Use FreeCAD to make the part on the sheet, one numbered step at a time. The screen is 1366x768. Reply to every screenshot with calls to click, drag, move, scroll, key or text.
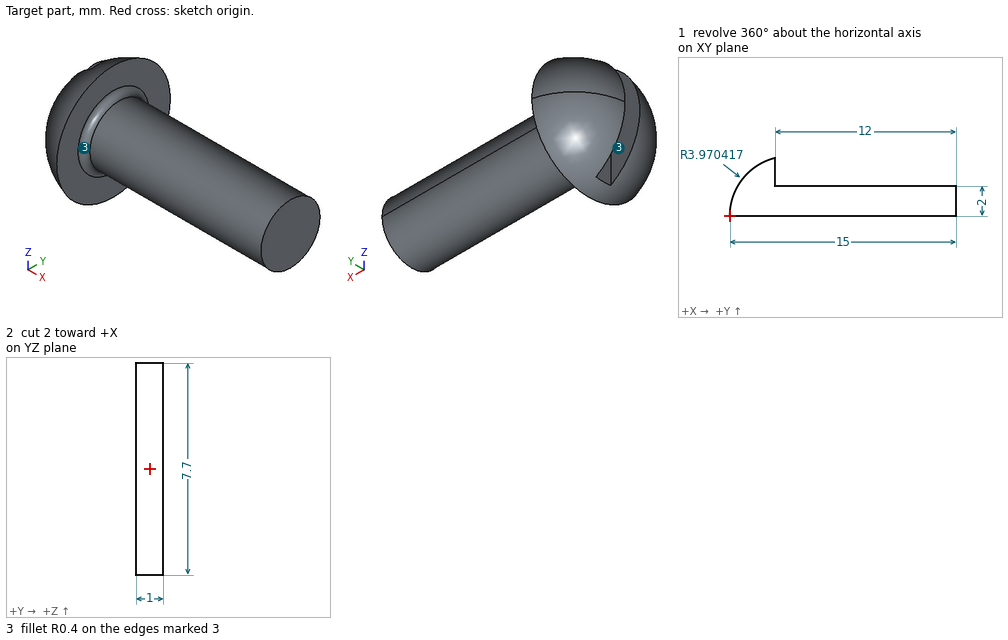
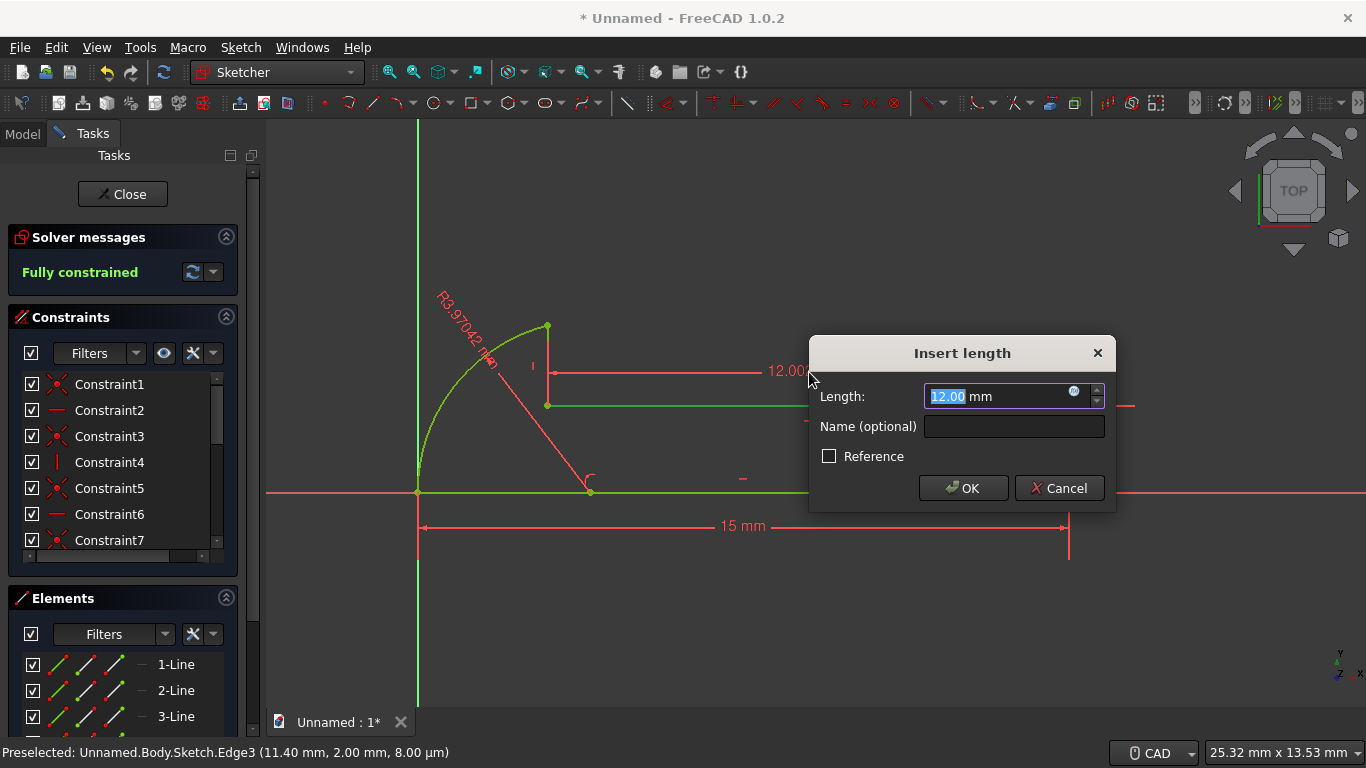
text(12)
key(Return)
key(Escape)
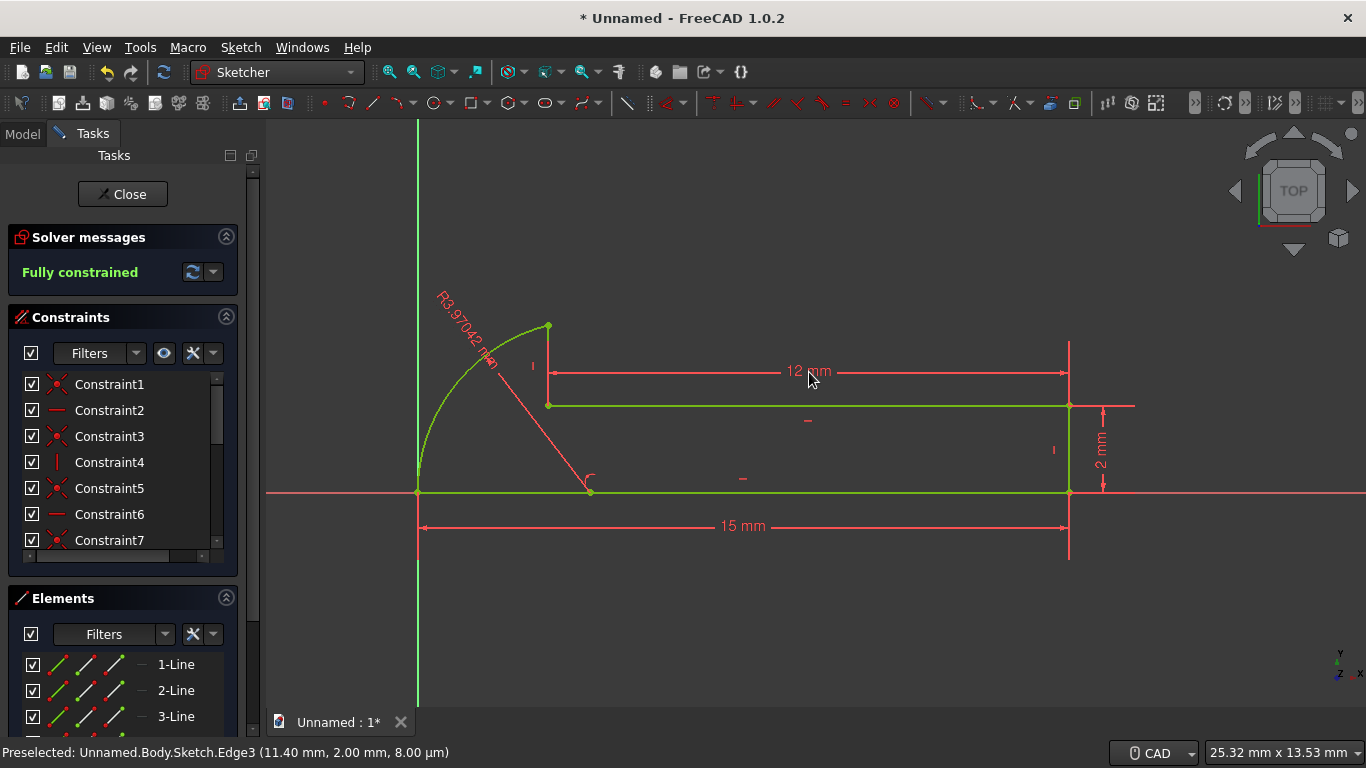
click(123, 194)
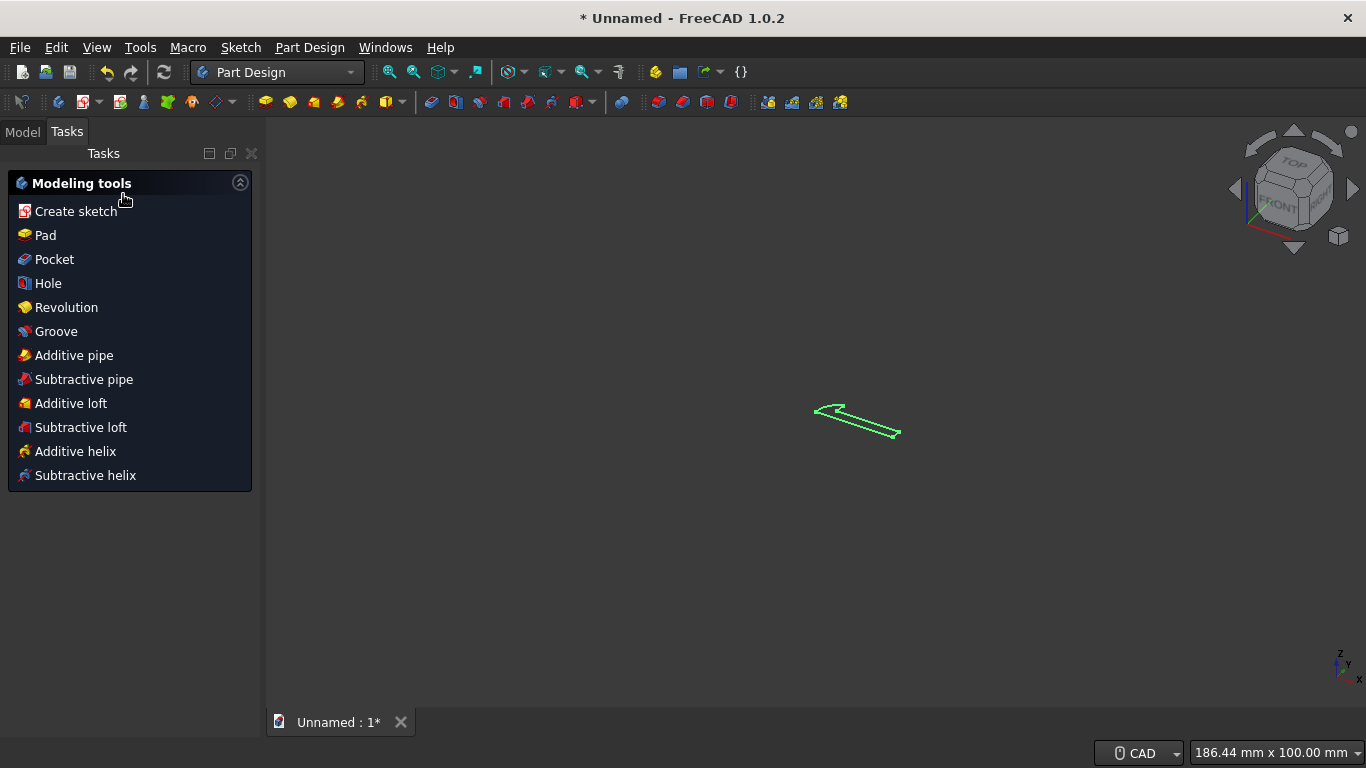
click(290, 102)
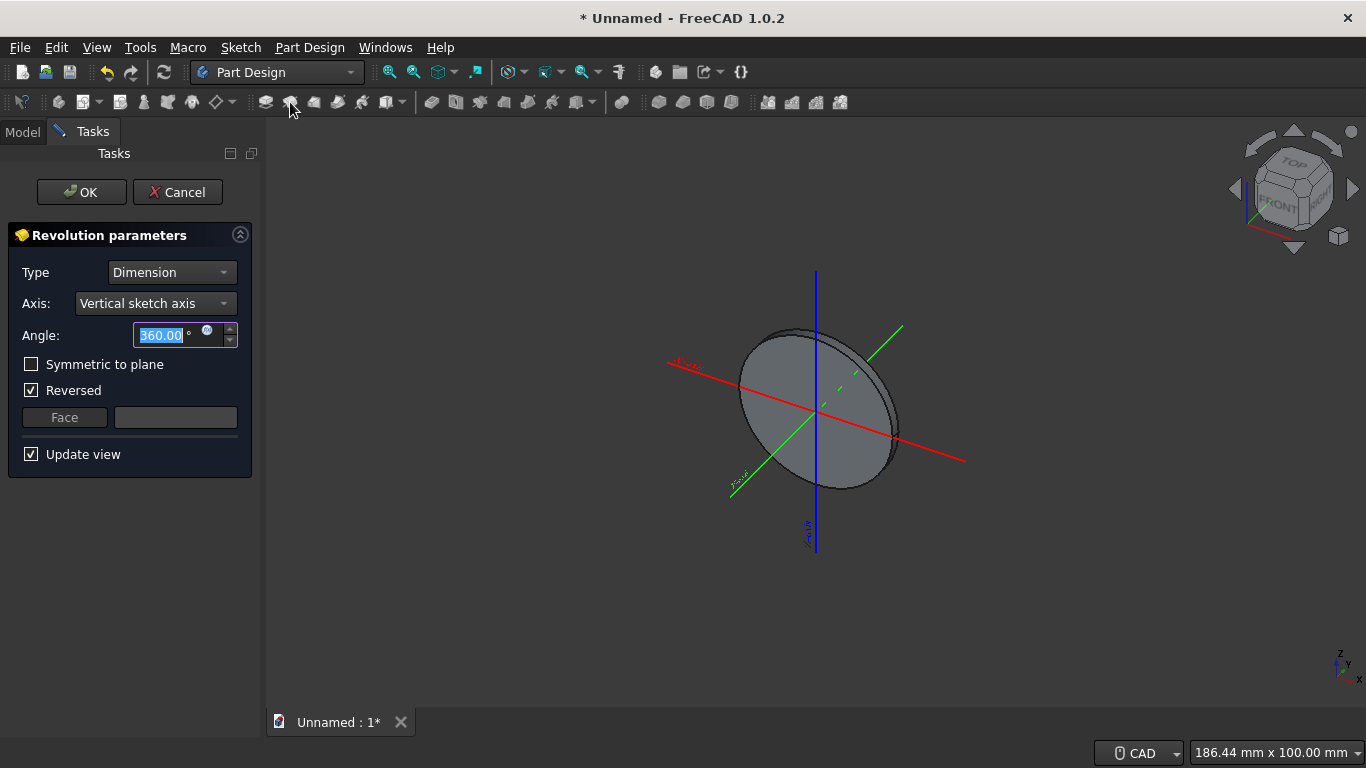
click(156, 304)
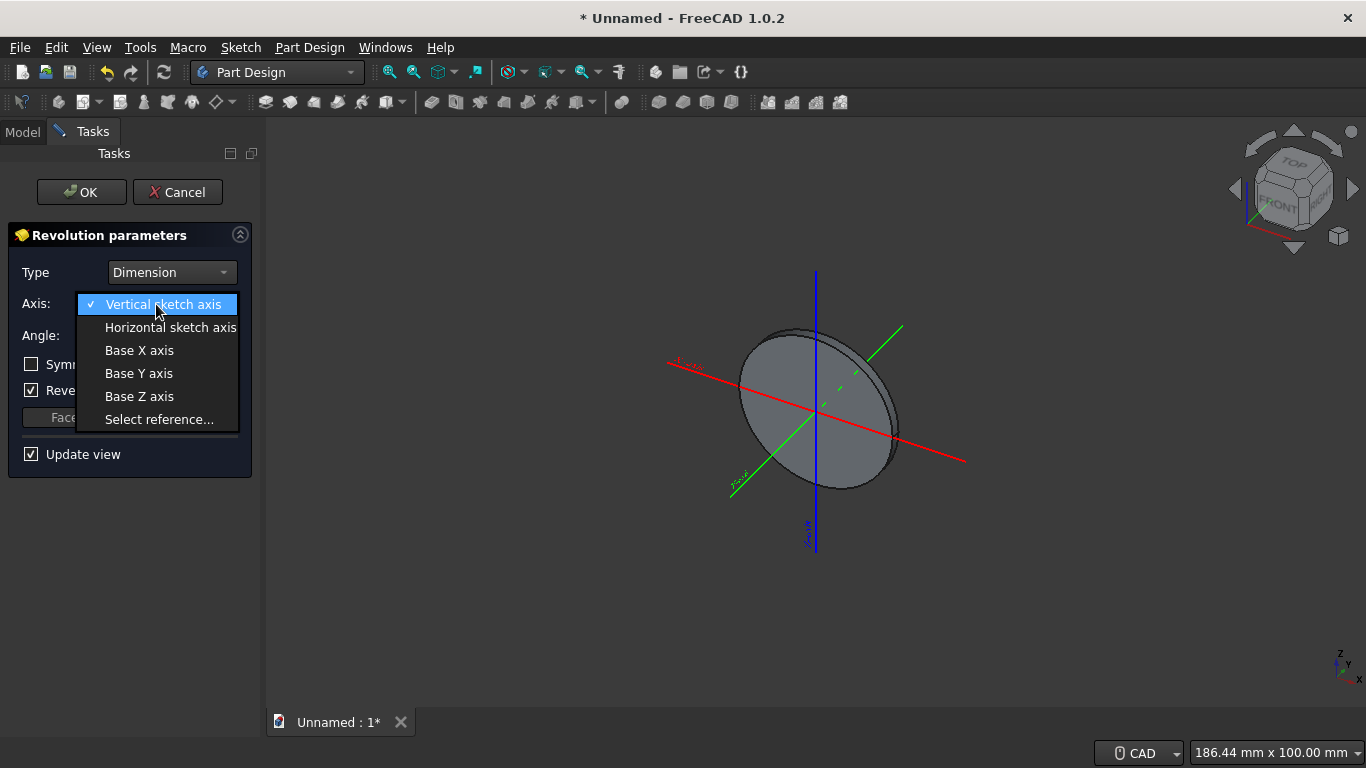
click(156, 328)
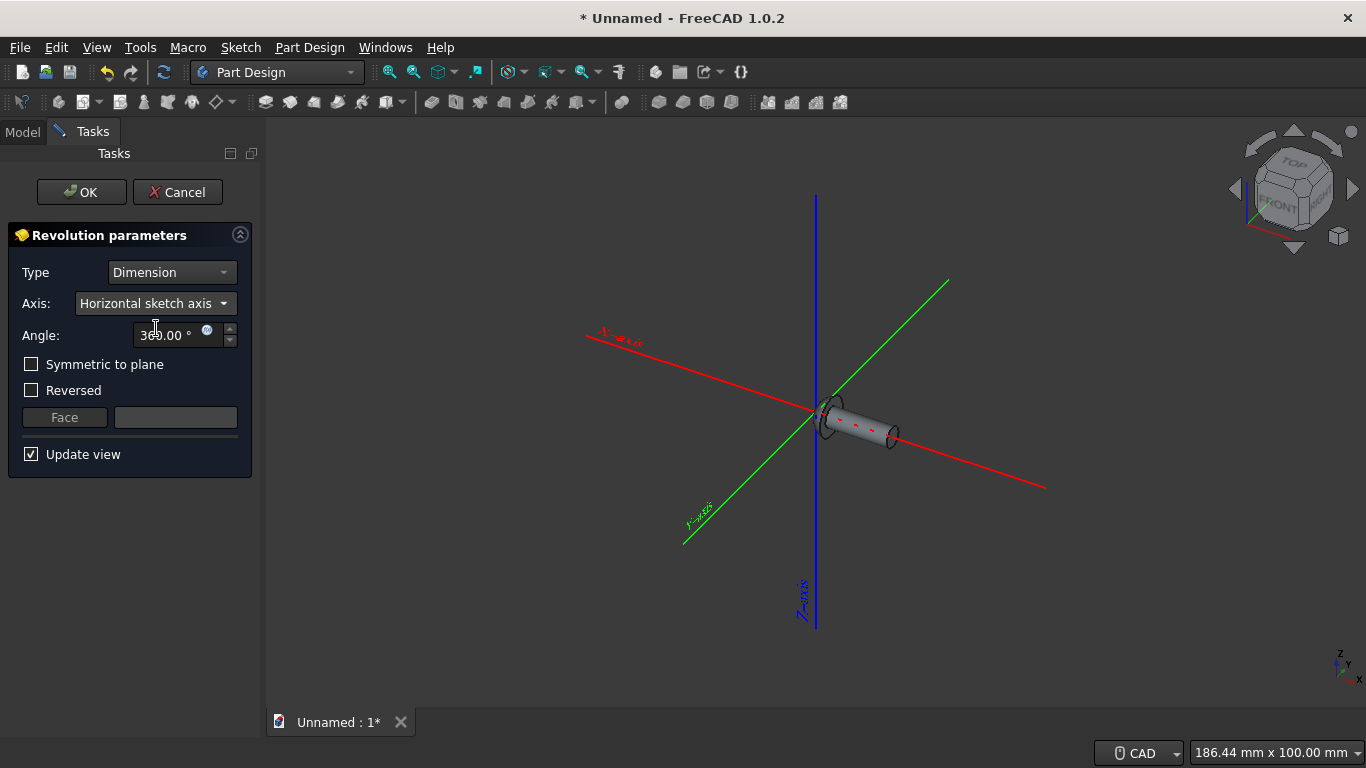
click(82, 192)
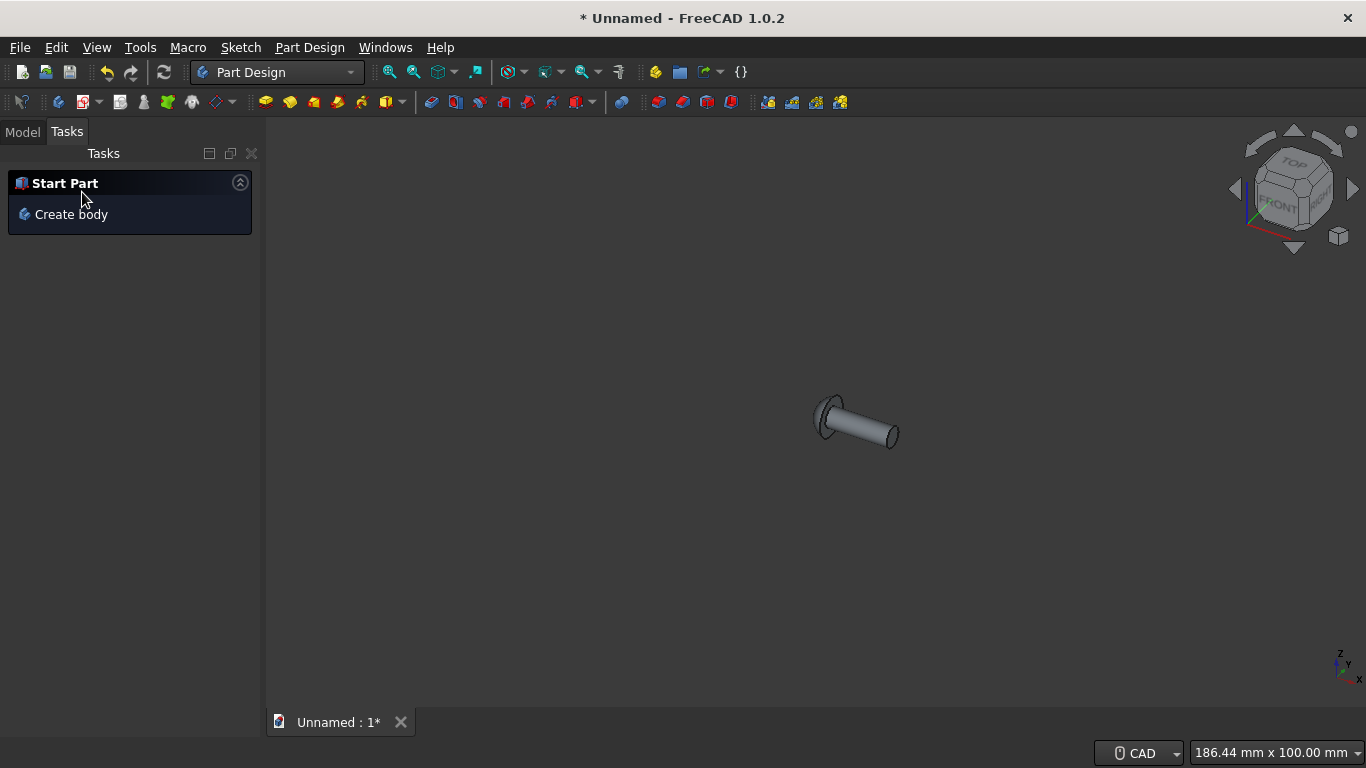
click(390, 72)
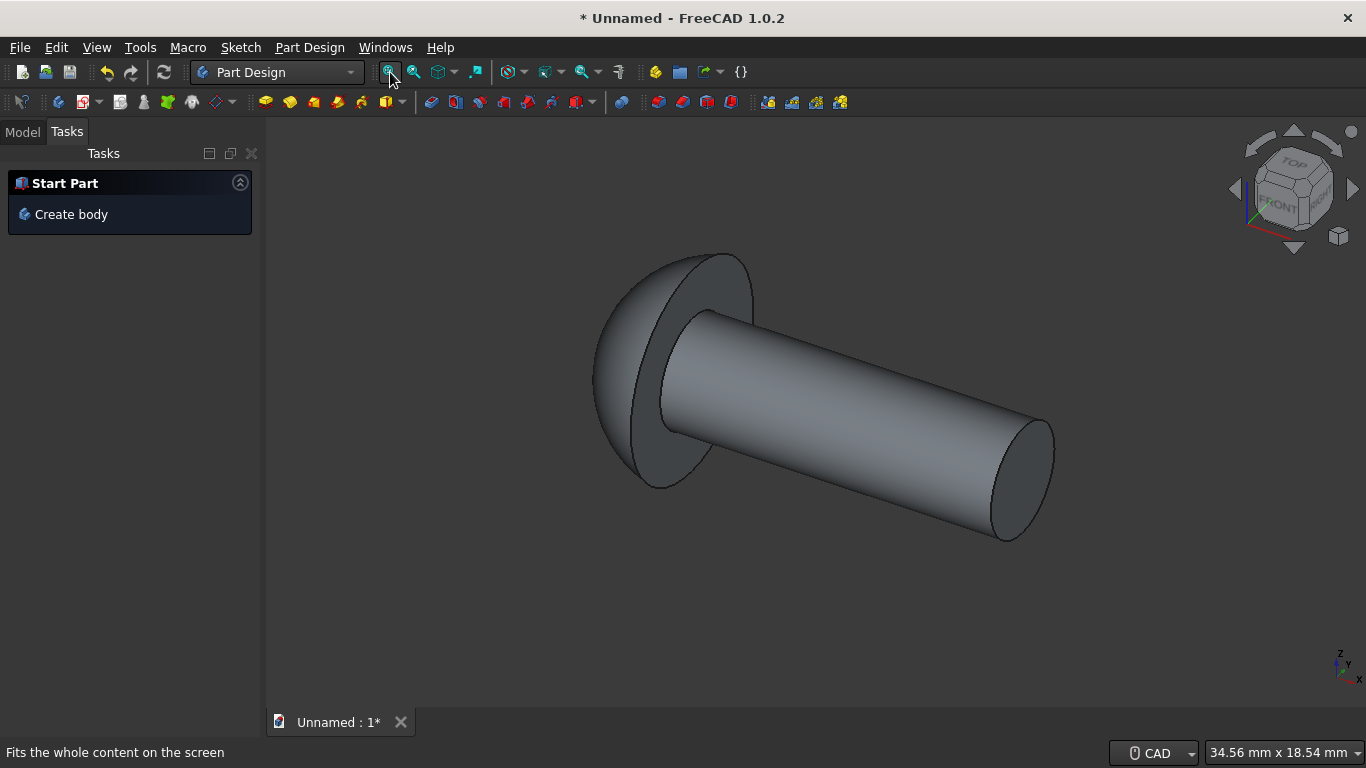
click(84, 102)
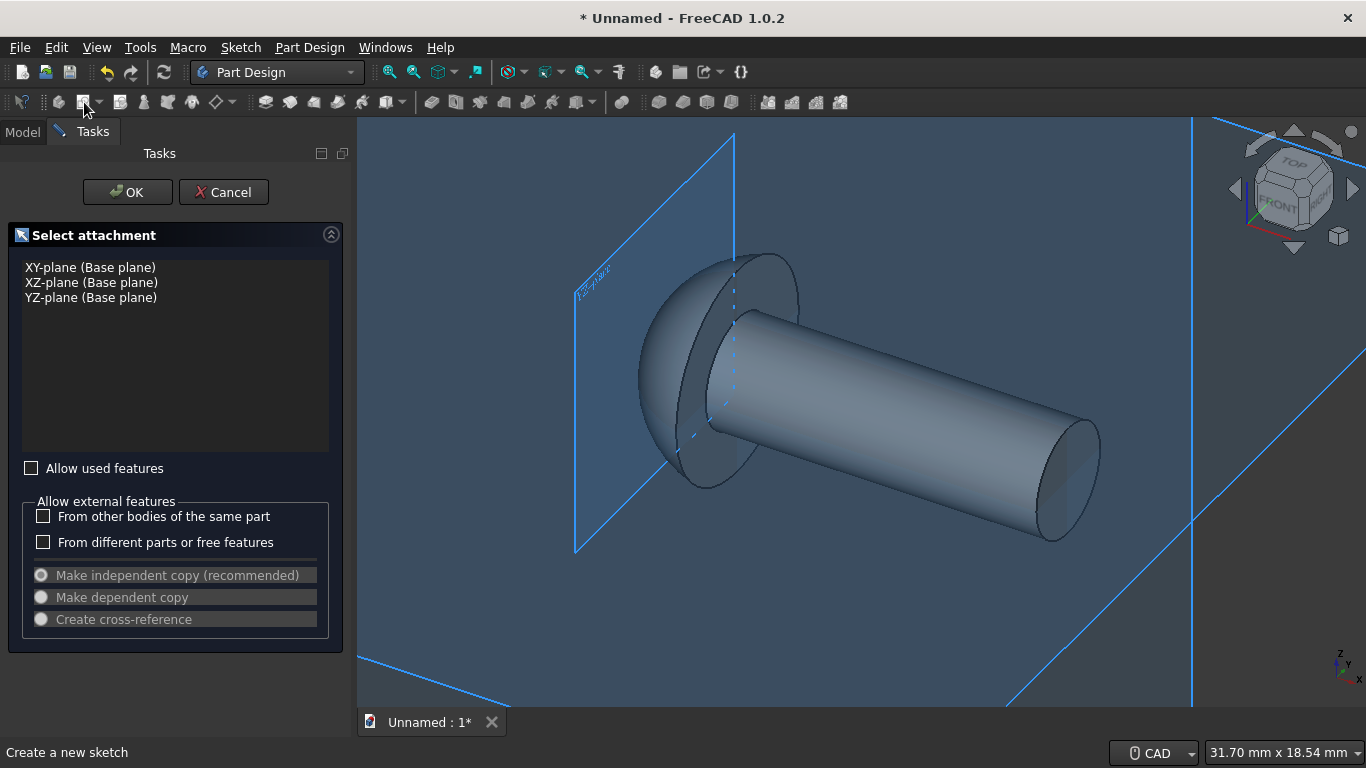
click(82, 298)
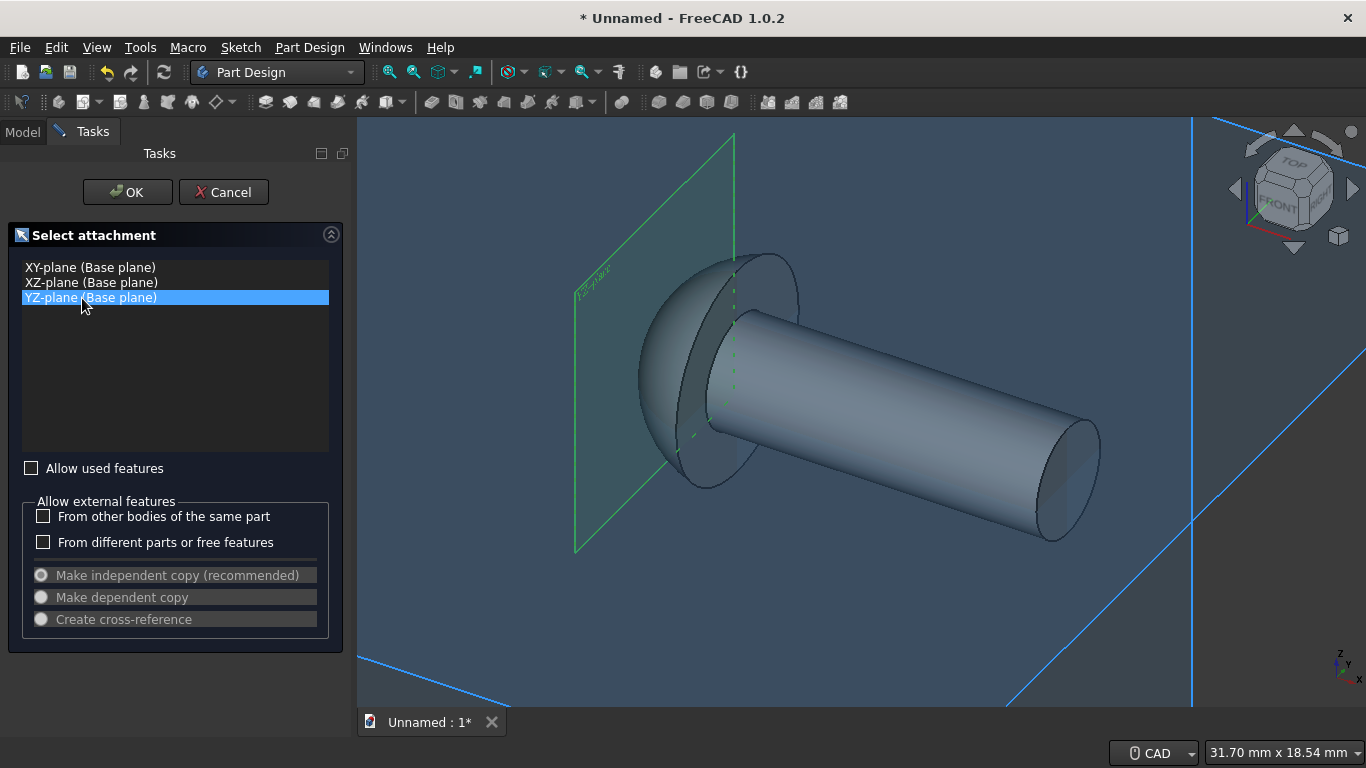
click(128, 192)